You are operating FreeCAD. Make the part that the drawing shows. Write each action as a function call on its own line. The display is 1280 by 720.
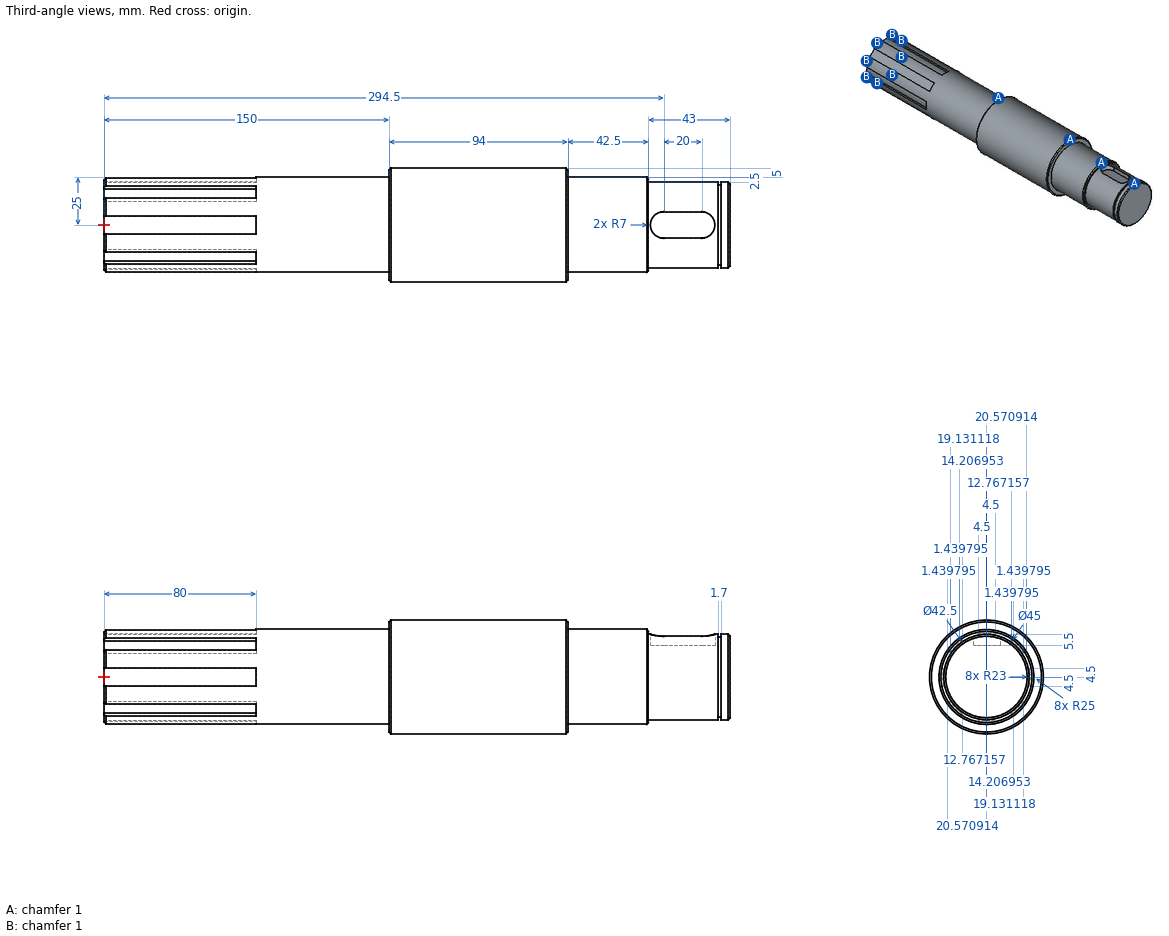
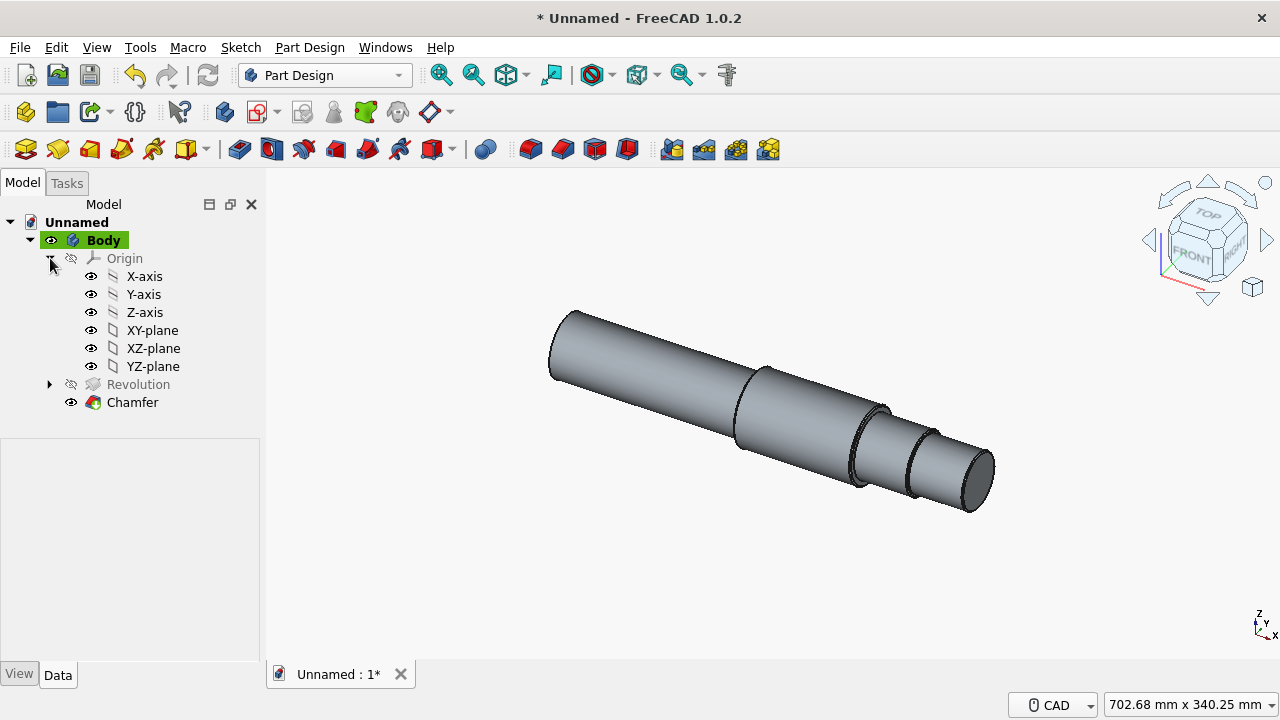
click(136, 366)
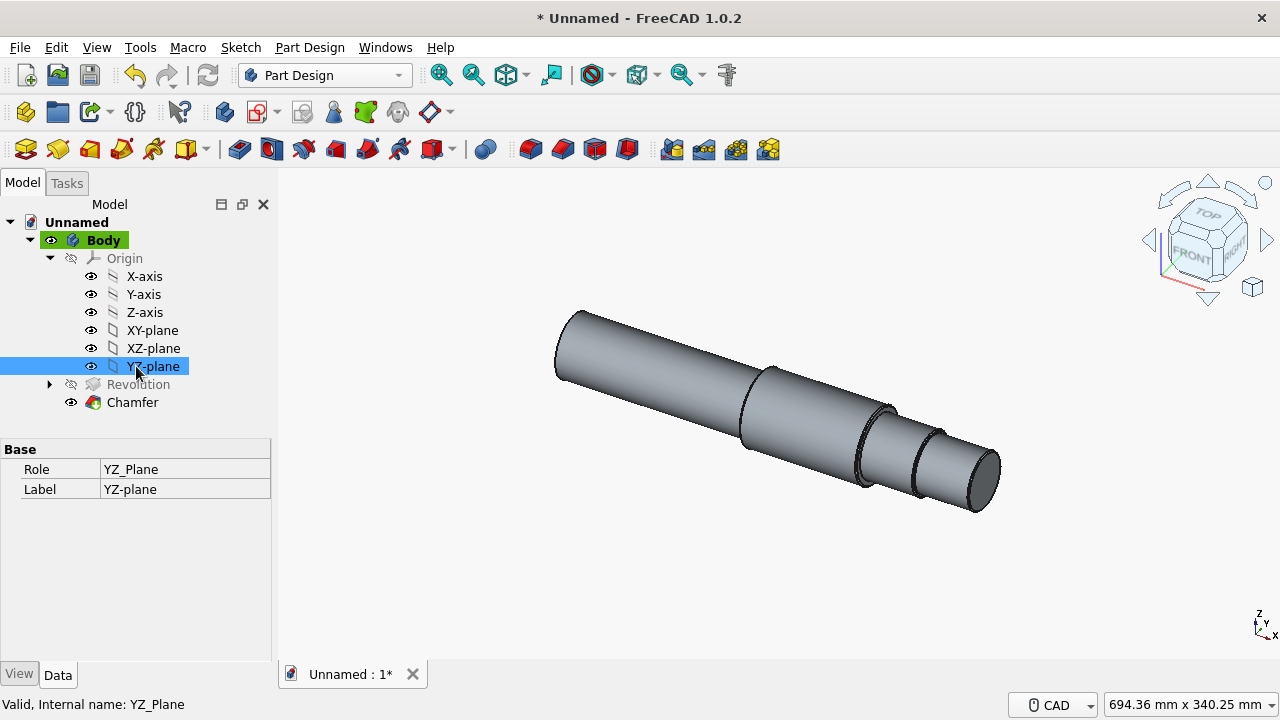
click(430, 112)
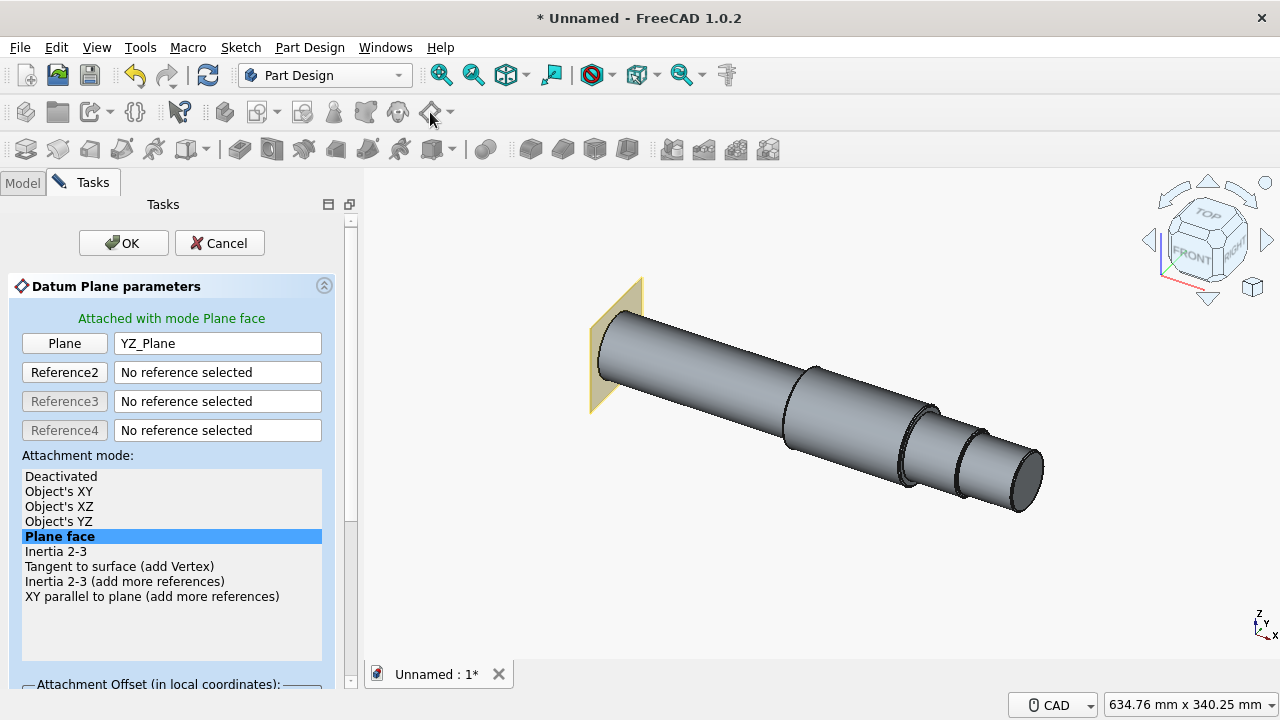
scroll(351, 451, down, 3)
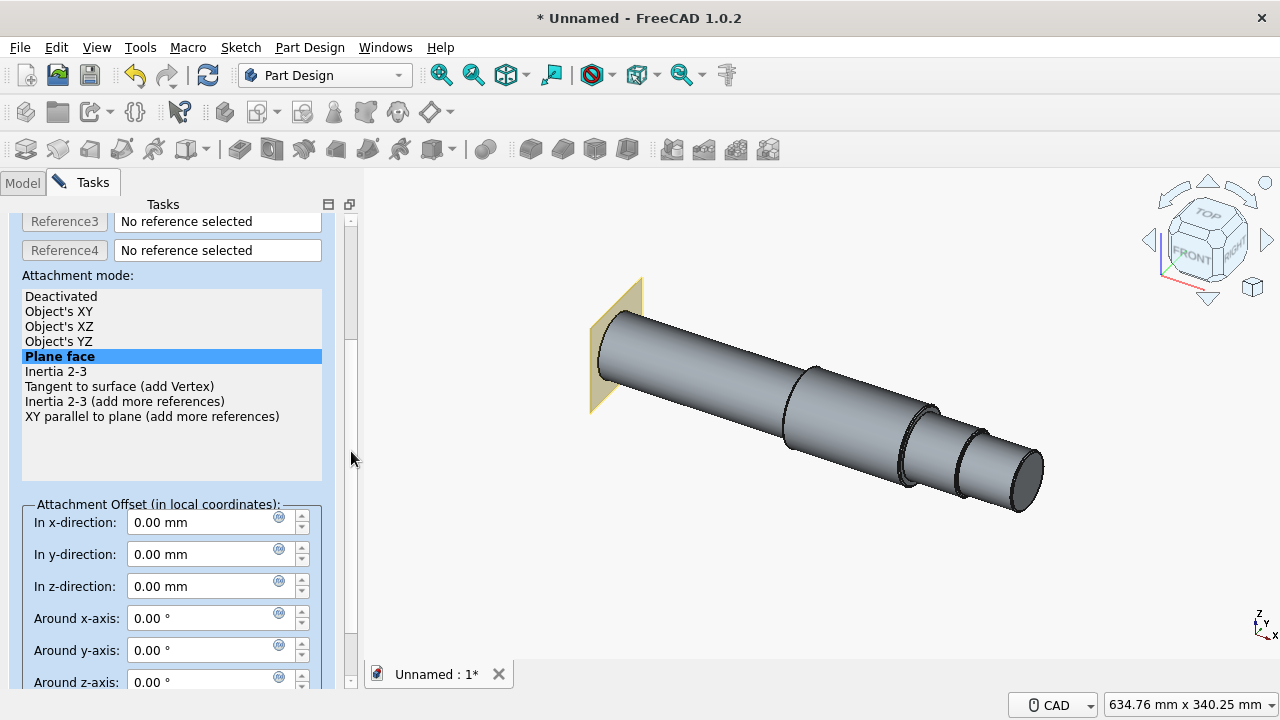
triple_click(210, 586)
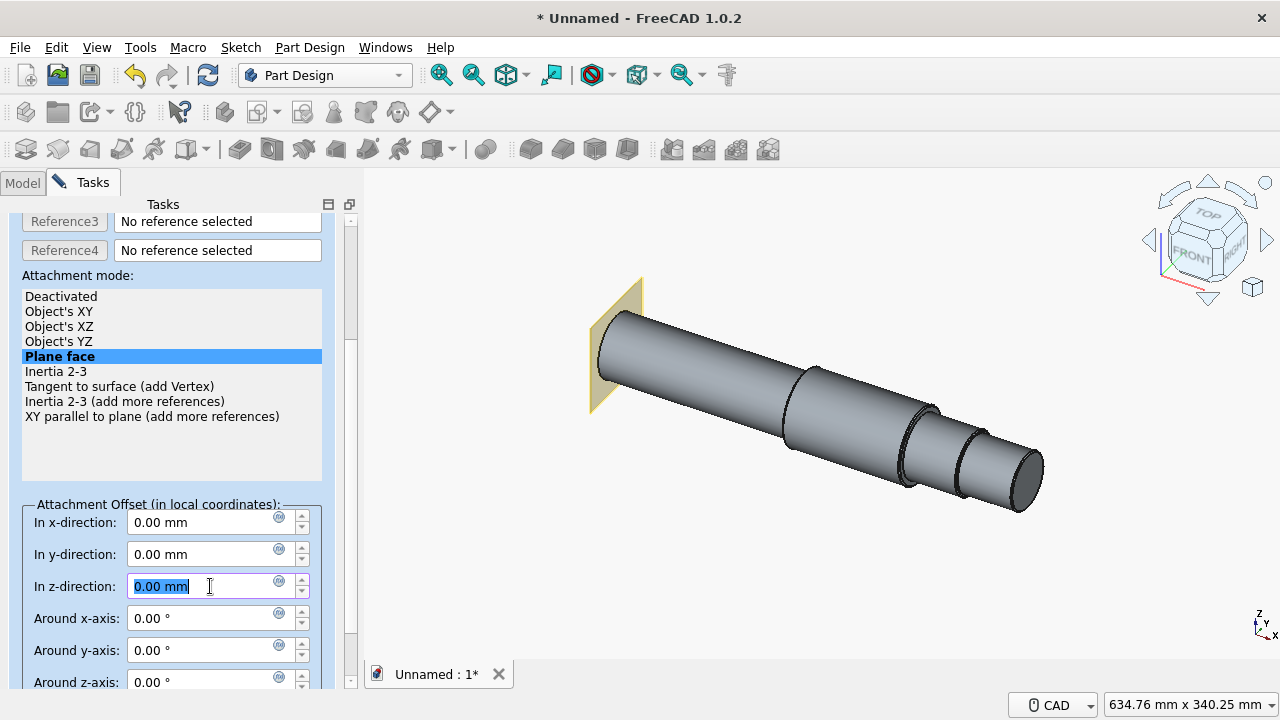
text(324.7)
key(Tab)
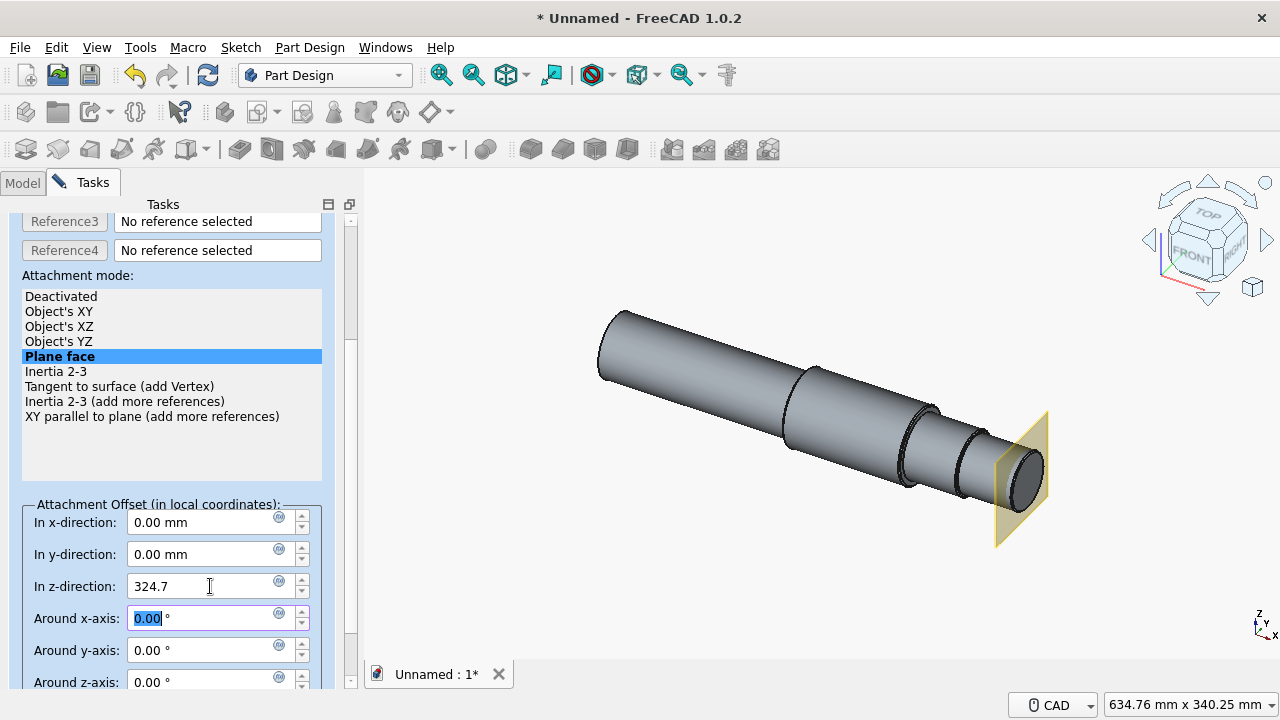
scroll(351, 451, up, 4)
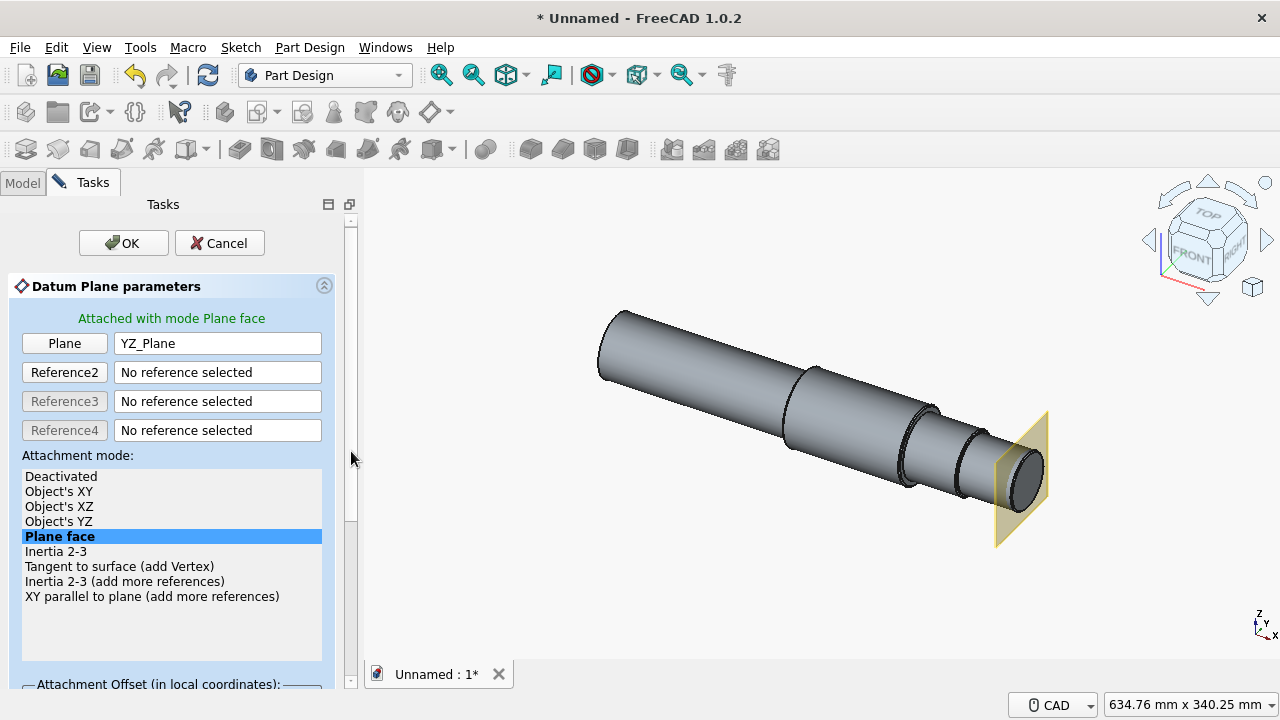
click(124, 243)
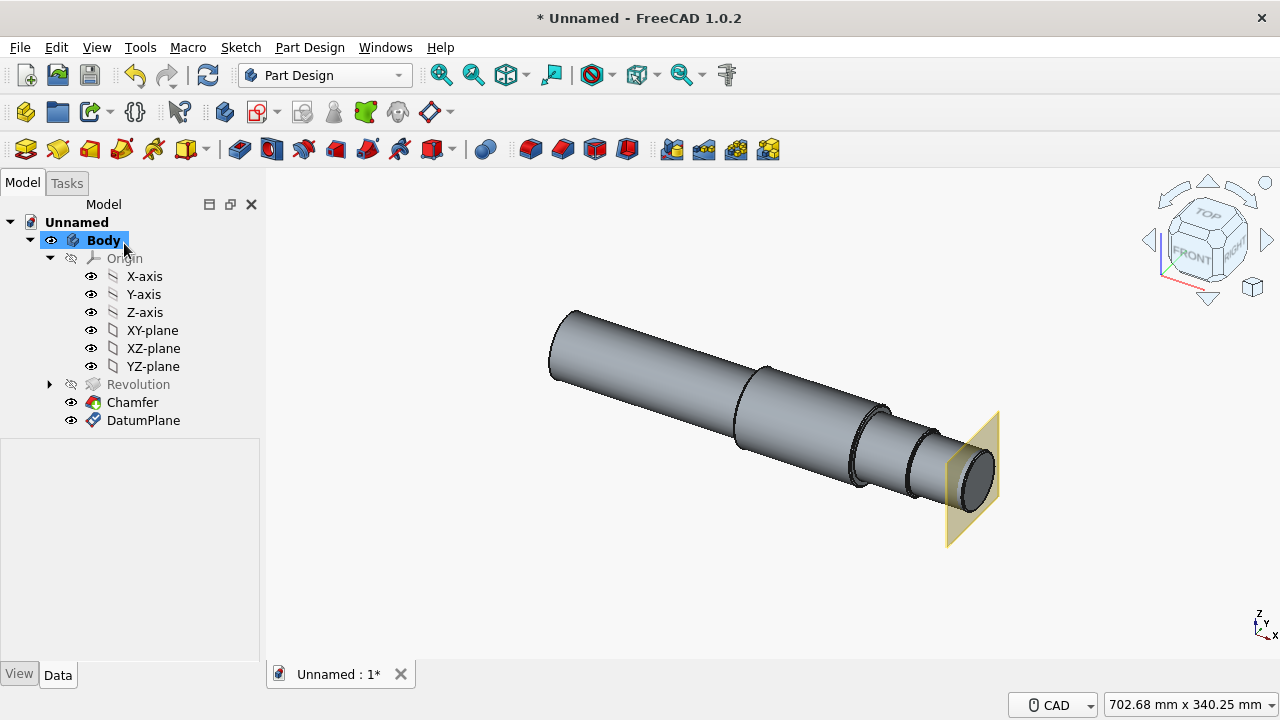
click(116, 420)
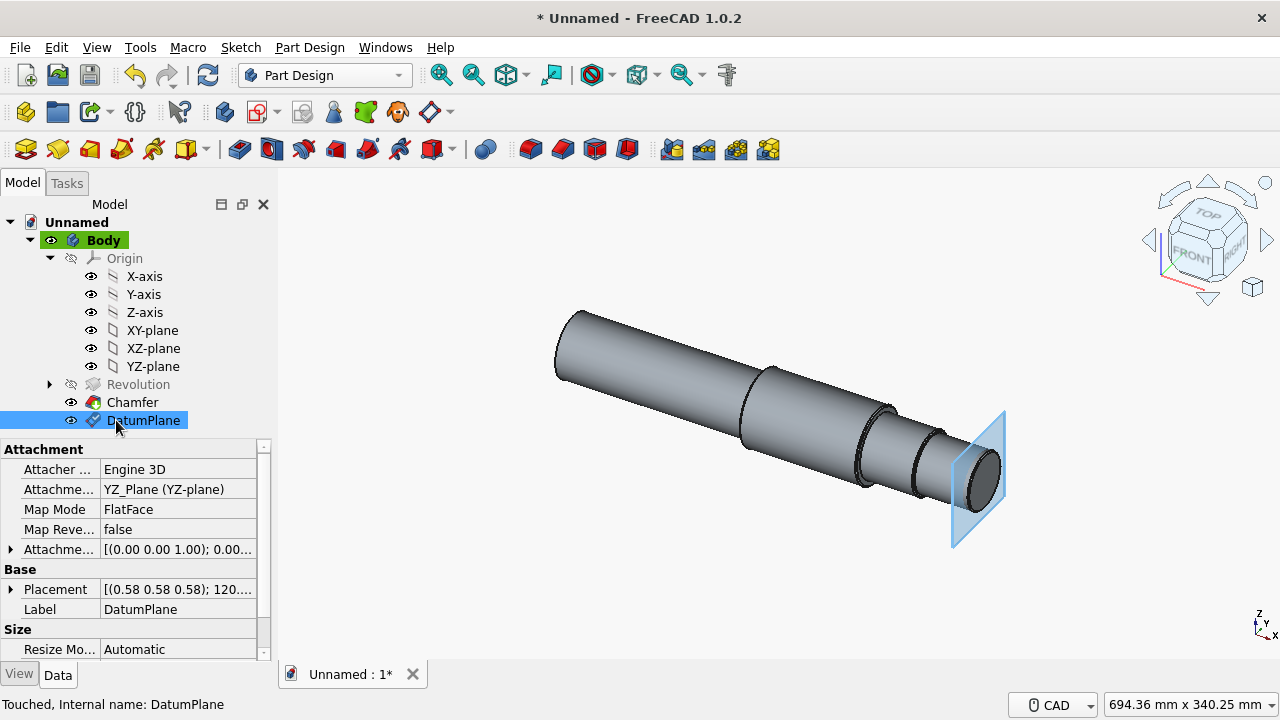
click(258, 112)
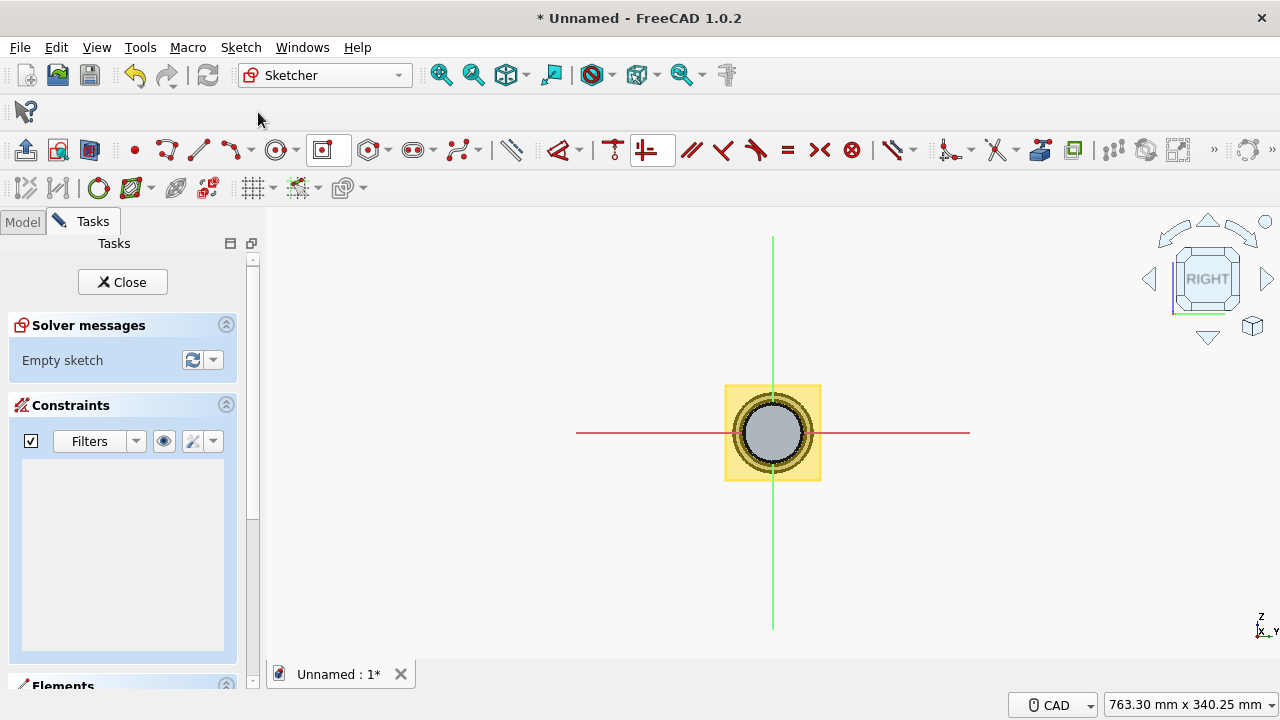
click(90, 150)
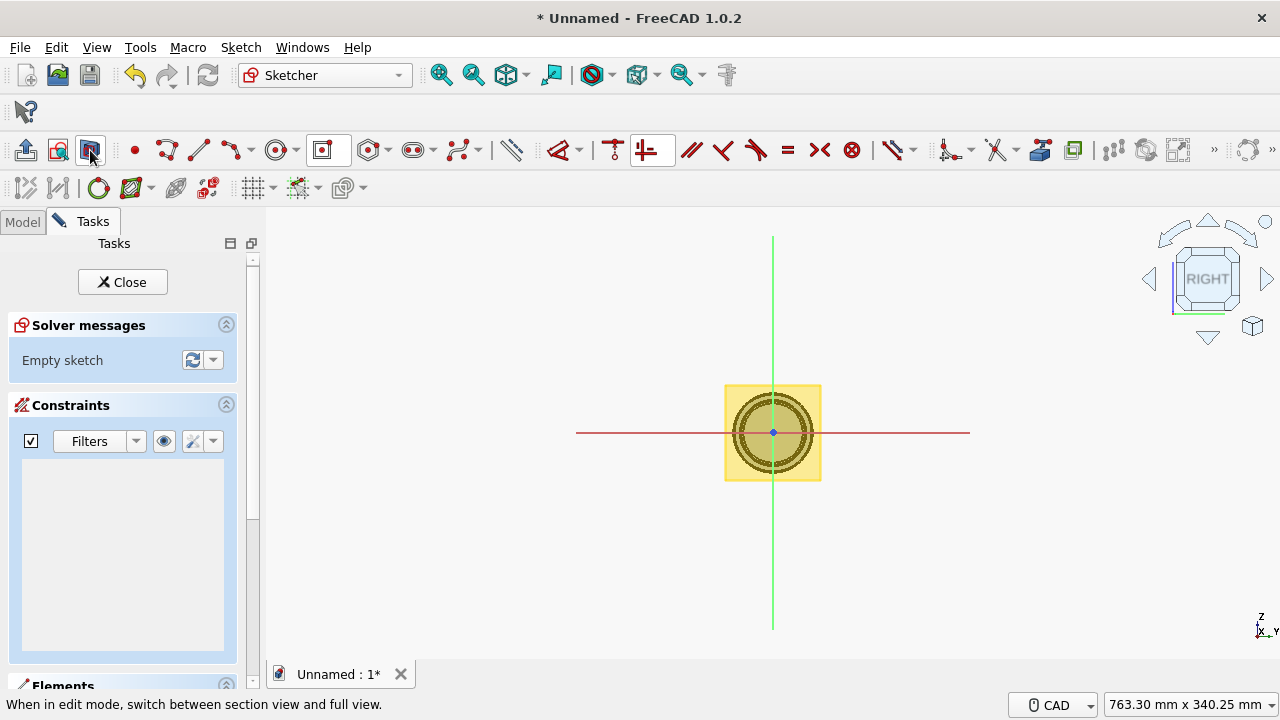
scroll(790, 433, up, 8)